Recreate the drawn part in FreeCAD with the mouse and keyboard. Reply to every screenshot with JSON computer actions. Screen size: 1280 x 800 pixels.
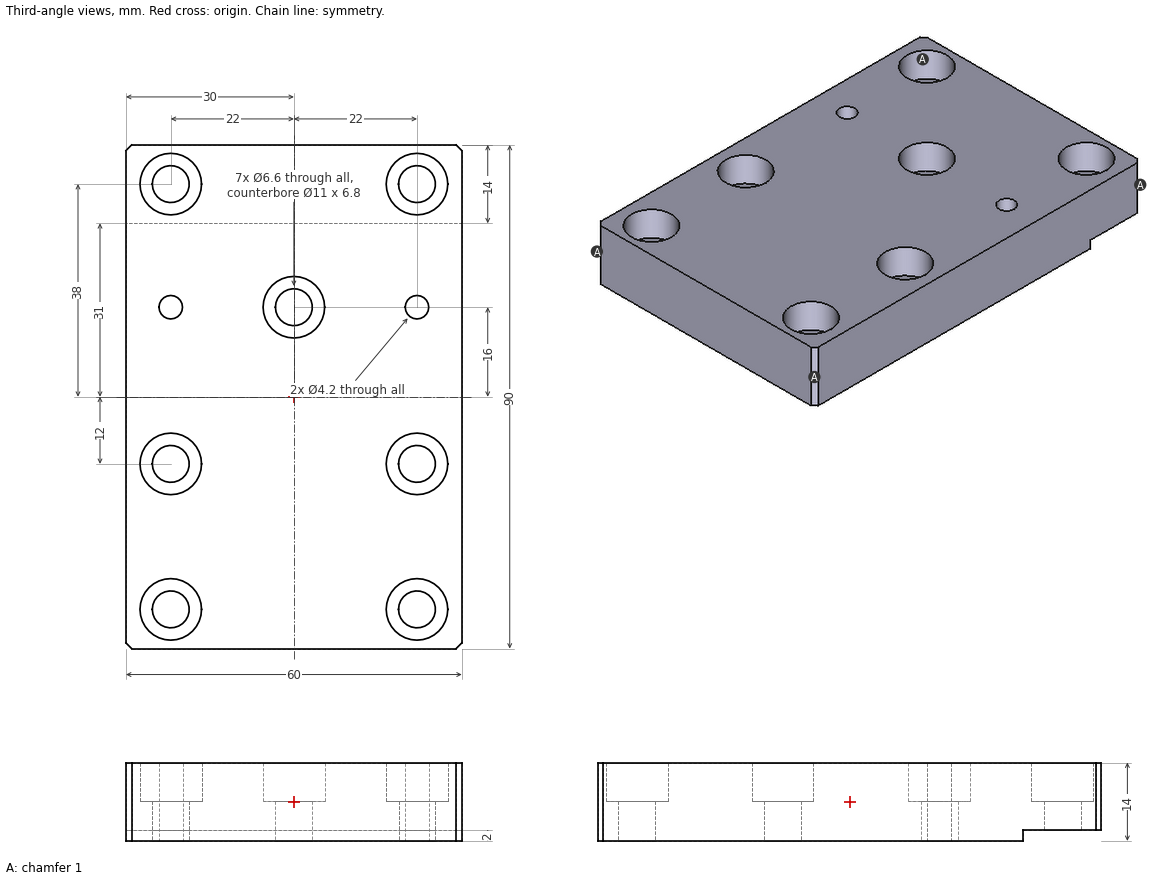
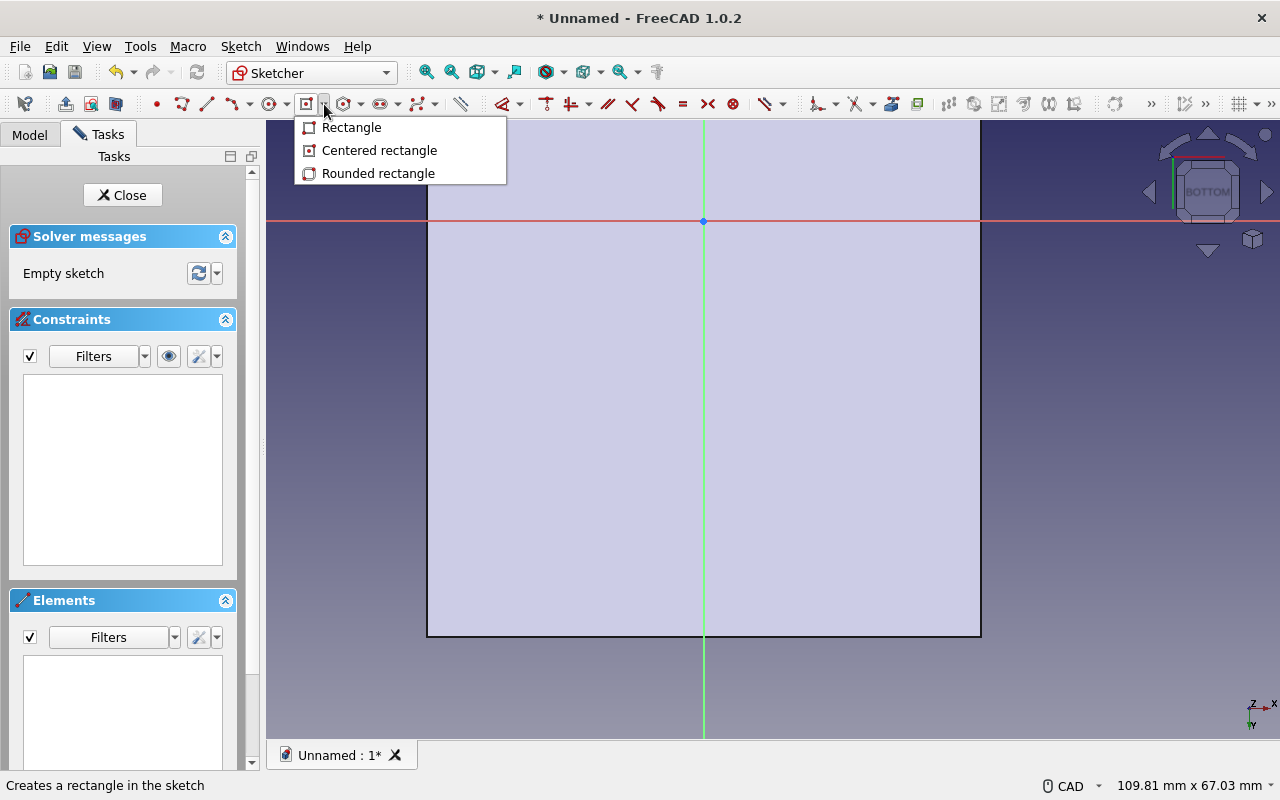
{"action": "left_click", "coordinate": [400, 128]}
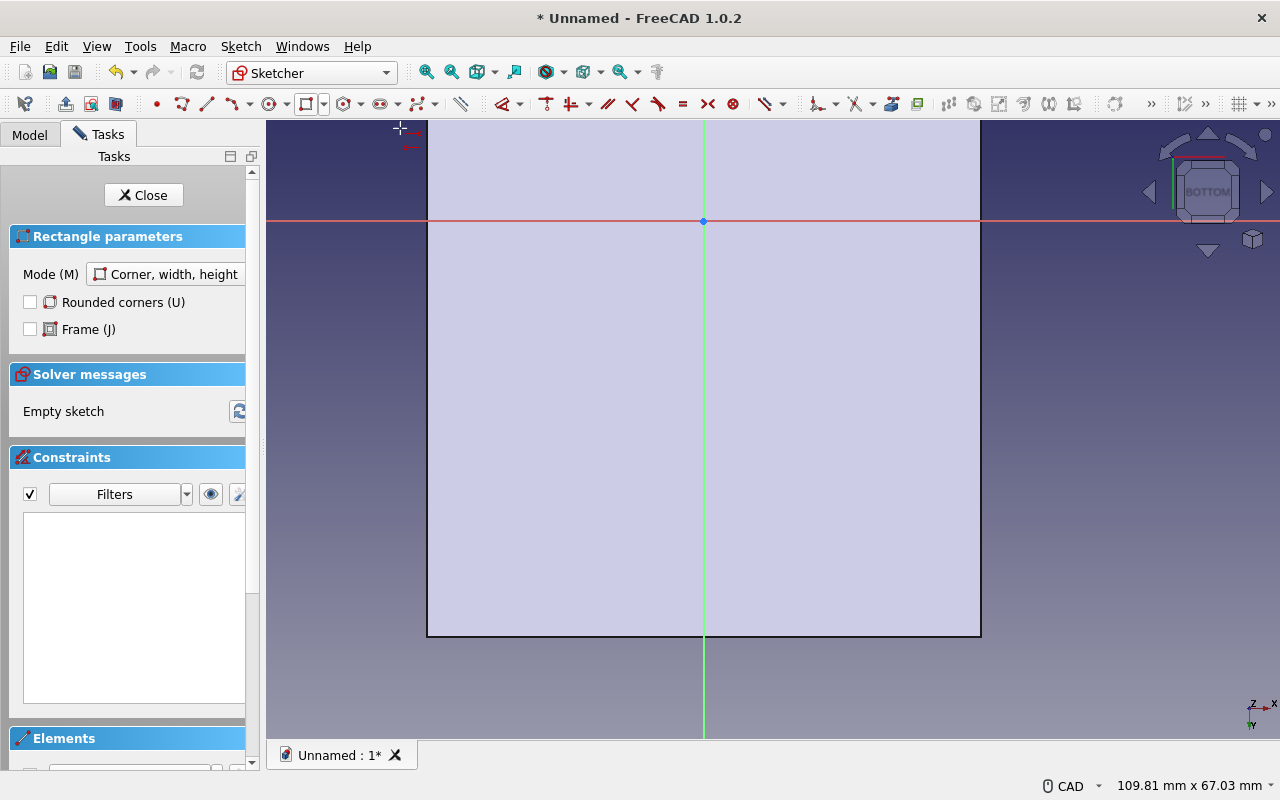
{"action": "left_click", "coordinate": [427, 508]}
{"action": "mouse_move", "coordinate": [981, 637]}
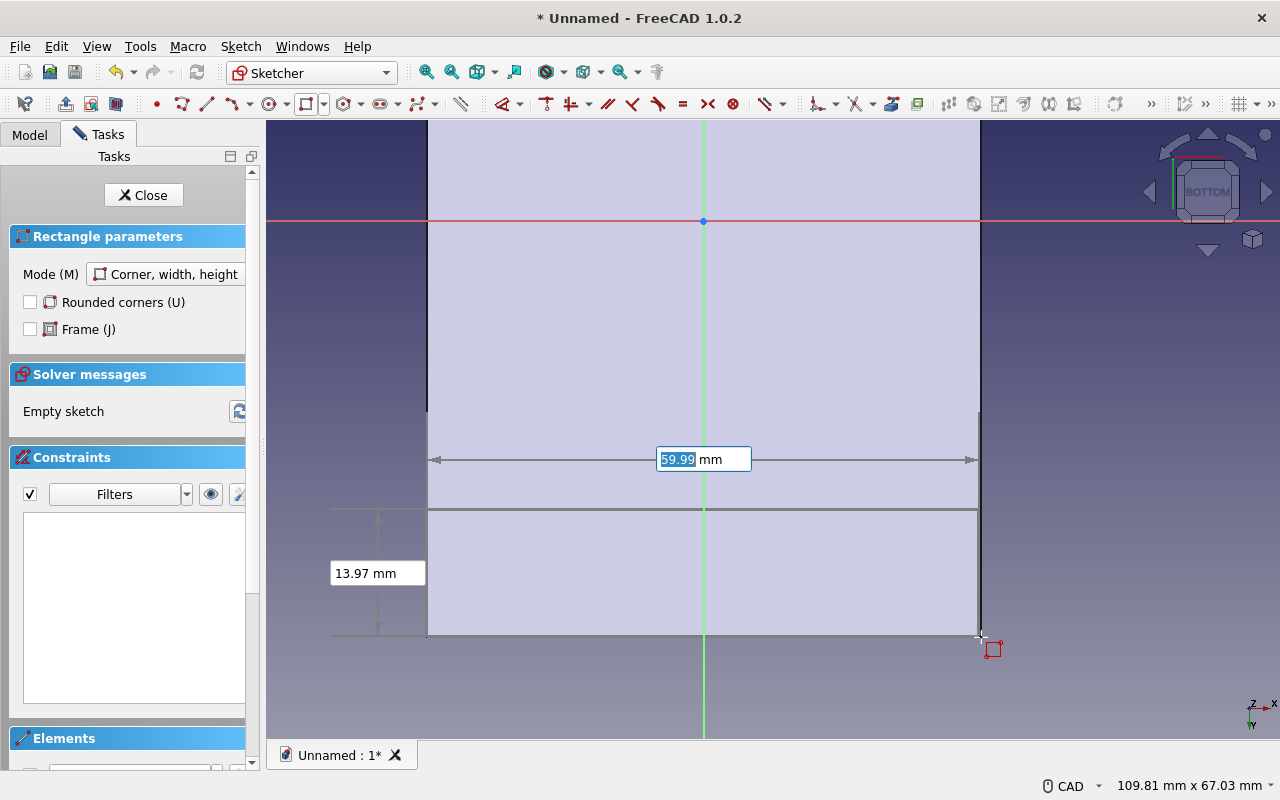
{"action": "type", "text": "60"}
{"action": "key", "text": "Tab"}
{"action": "type", "text": "14"}
{"action": "key", "text": "Return"}
{"action": "key", "text": "Escape"}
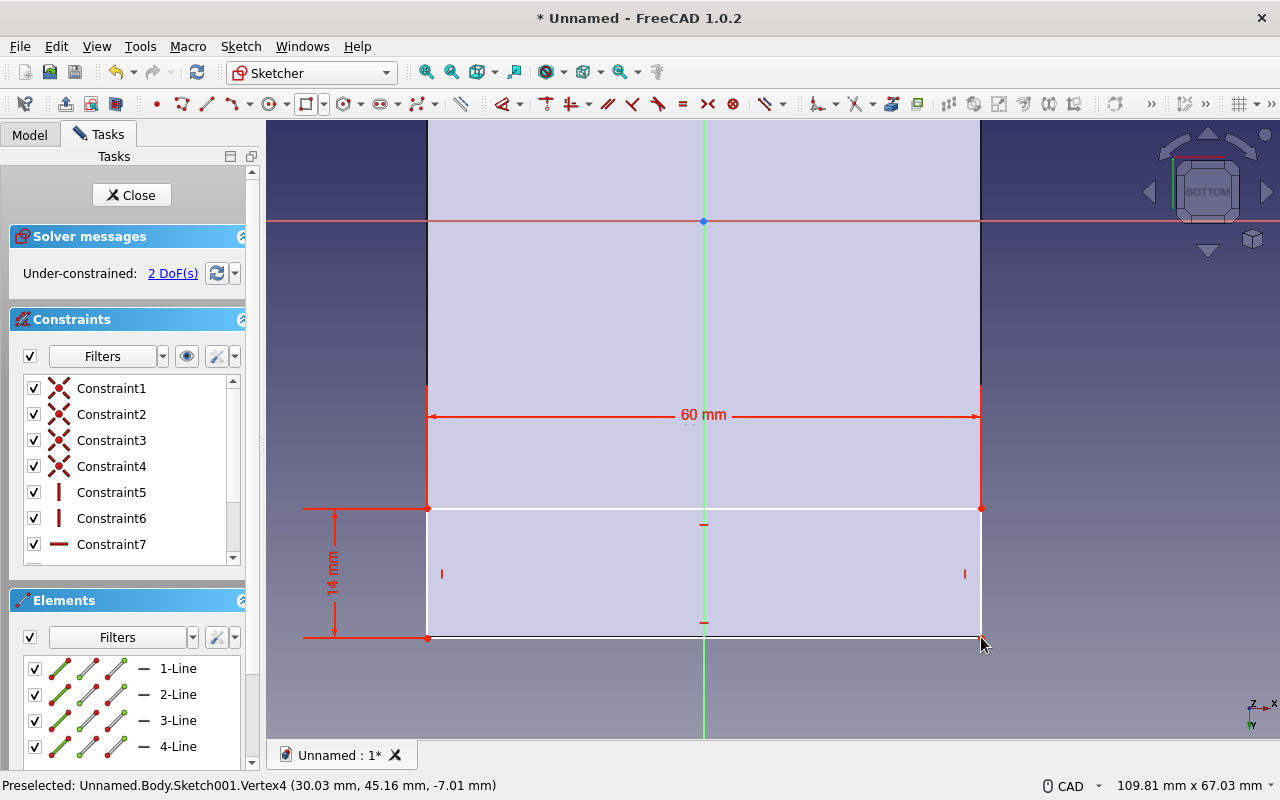
{"action": "left_click", "coordinate": [427, 509]}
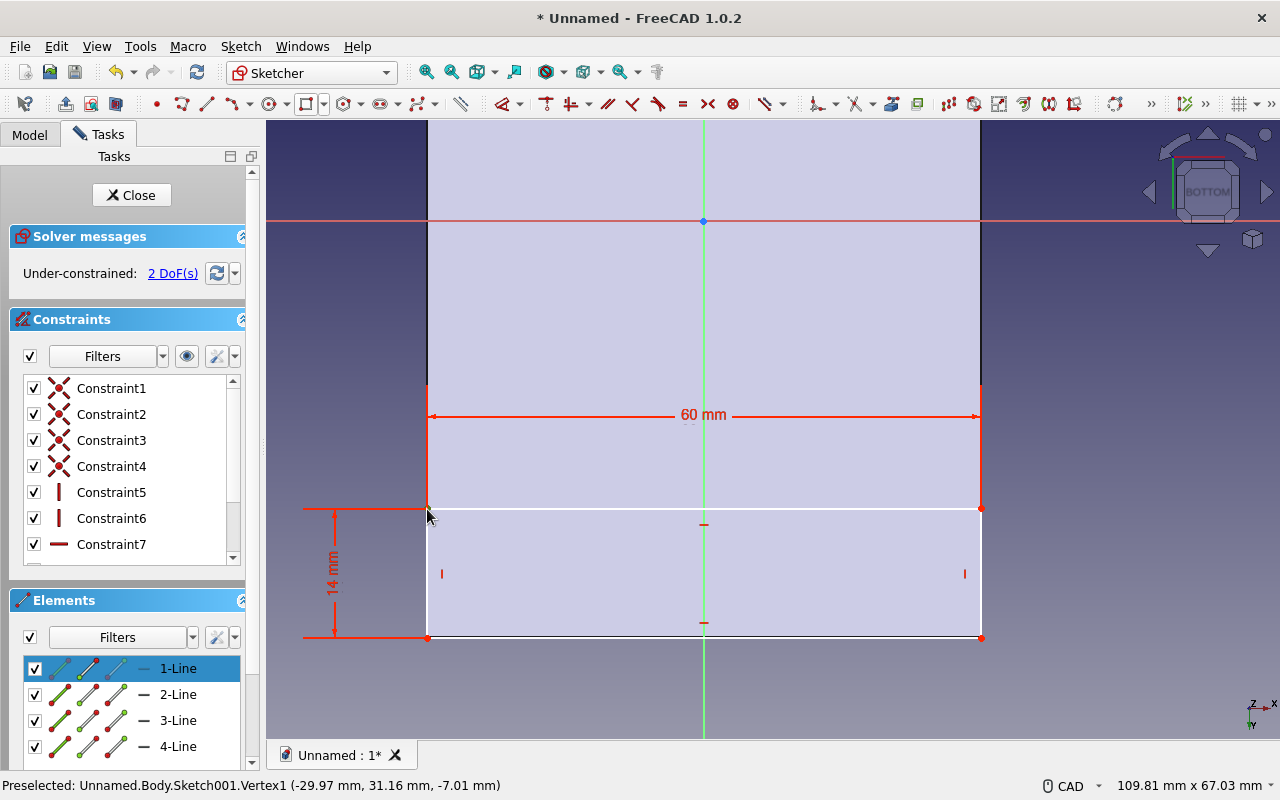
{"action": "left_click", "coordinate": [520, 104]}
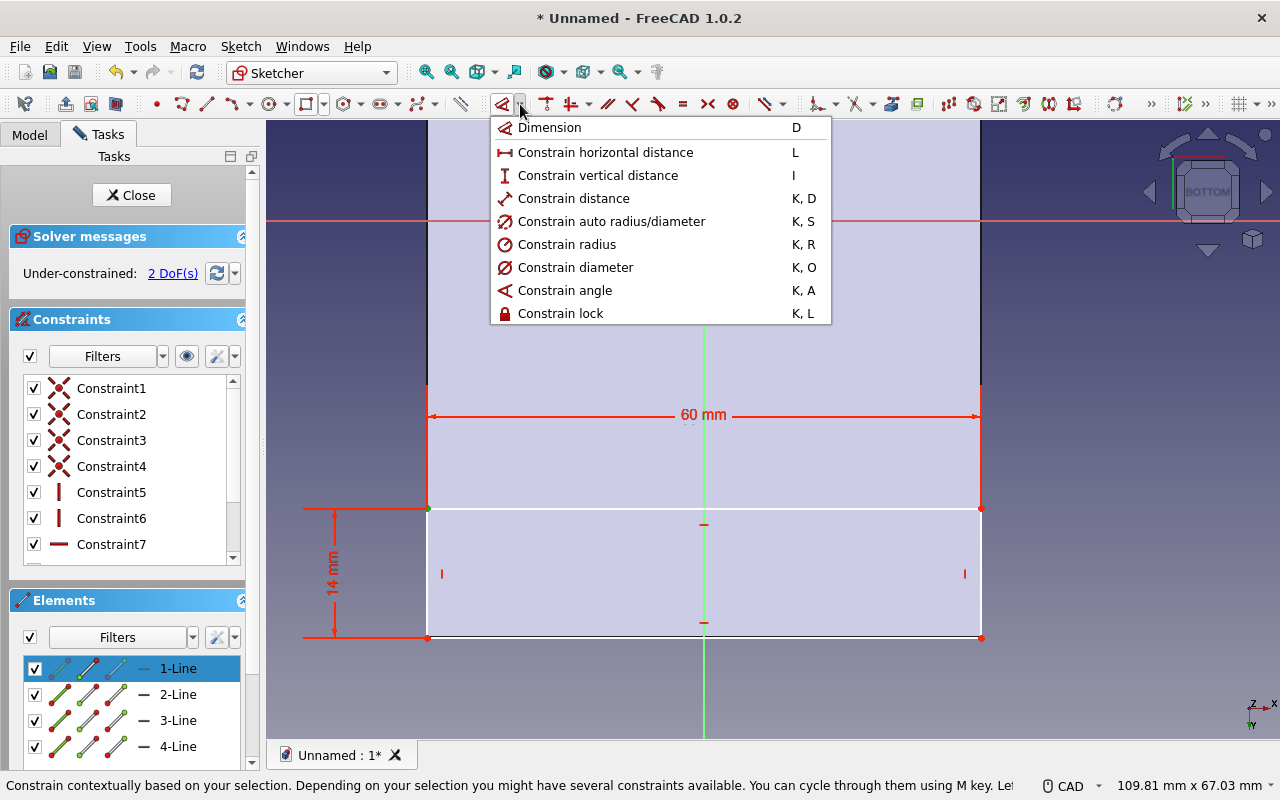
{"action": "left_click", "coordinate": [661, 152]}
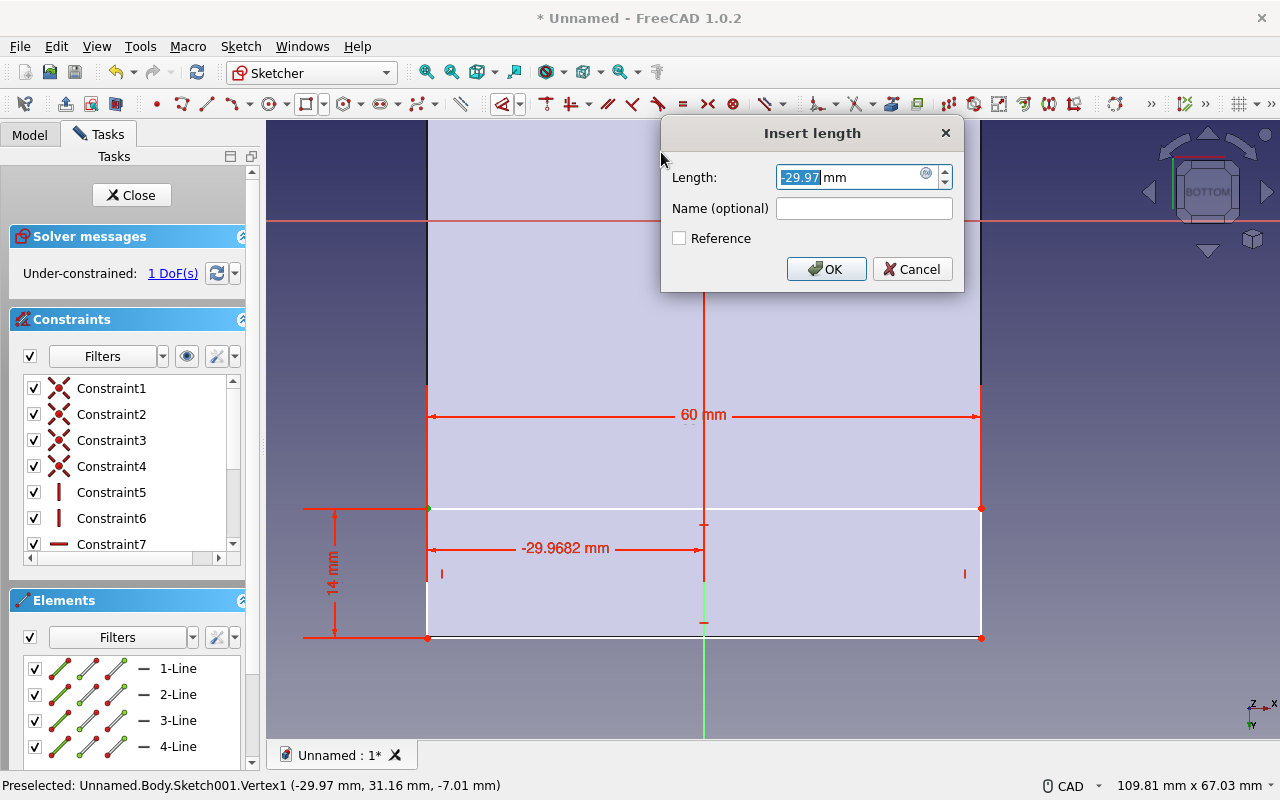
{"action": "type", "text": "-30"}
{"action": "key", "text": "Return"}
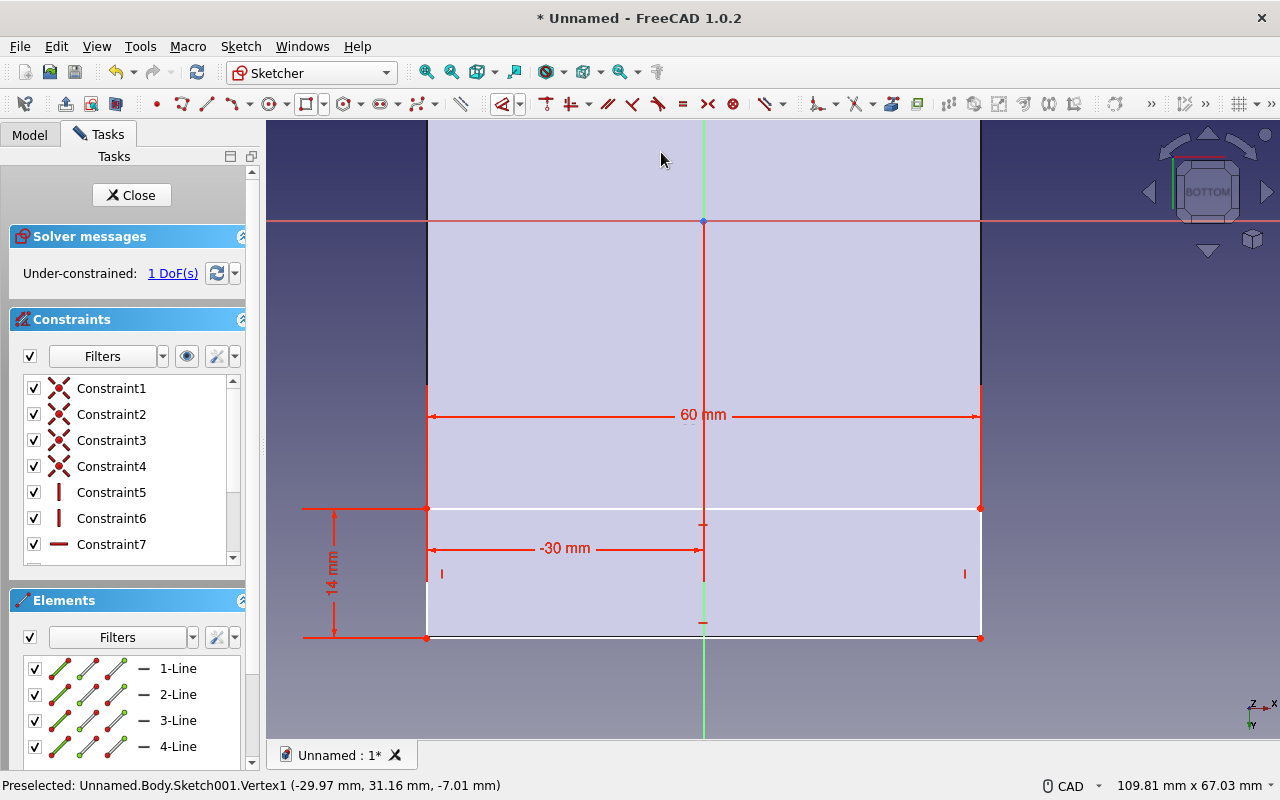
{"action": "left_click", "coordinate": [427, 509]}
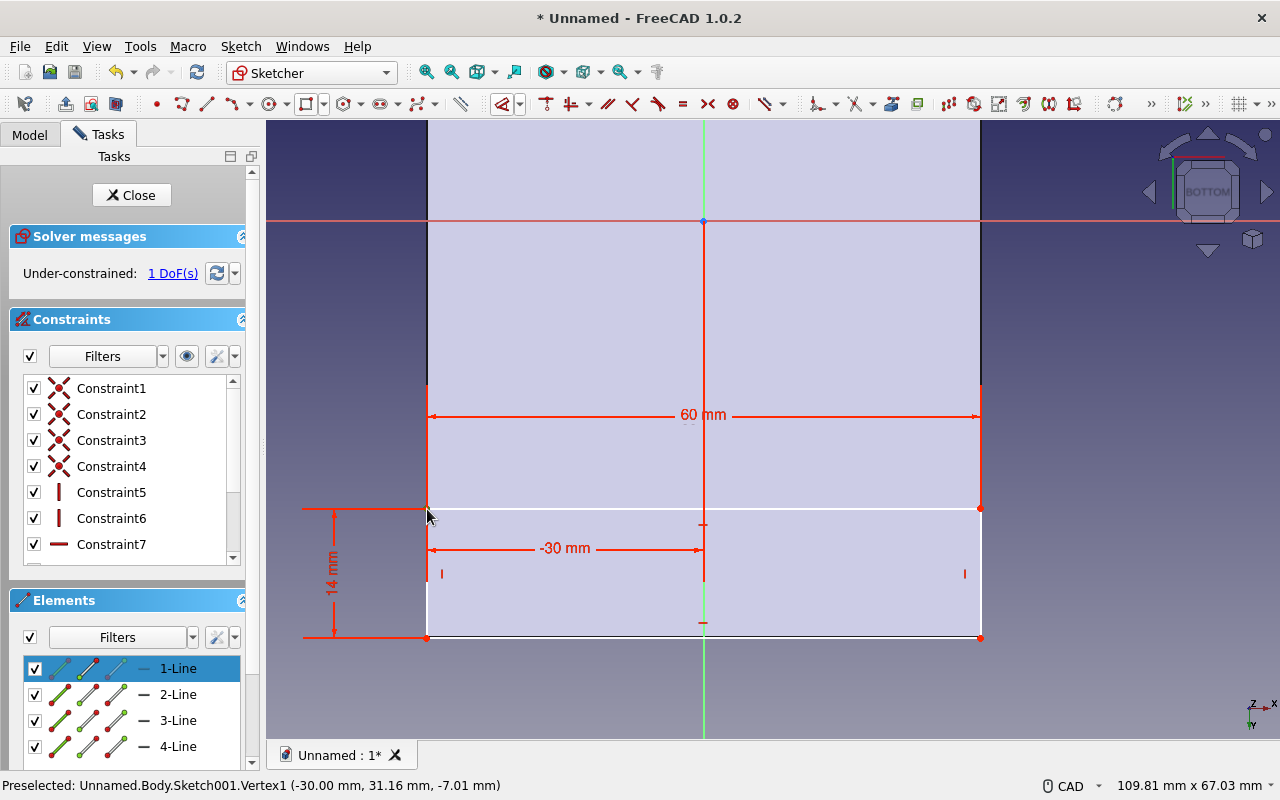
{"action": "left_click", "coordinate": [520, 104]}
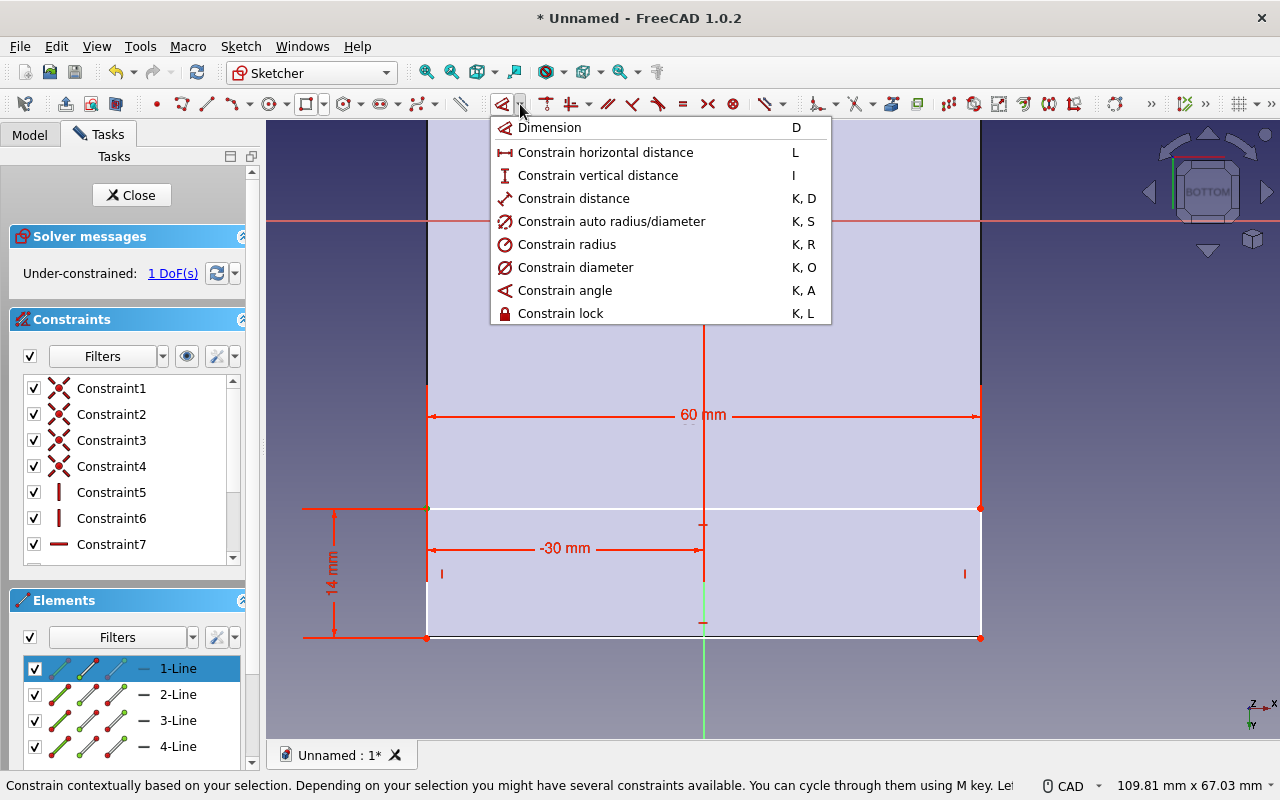
{"action": "left_click", "coordinate": [661, 176]}